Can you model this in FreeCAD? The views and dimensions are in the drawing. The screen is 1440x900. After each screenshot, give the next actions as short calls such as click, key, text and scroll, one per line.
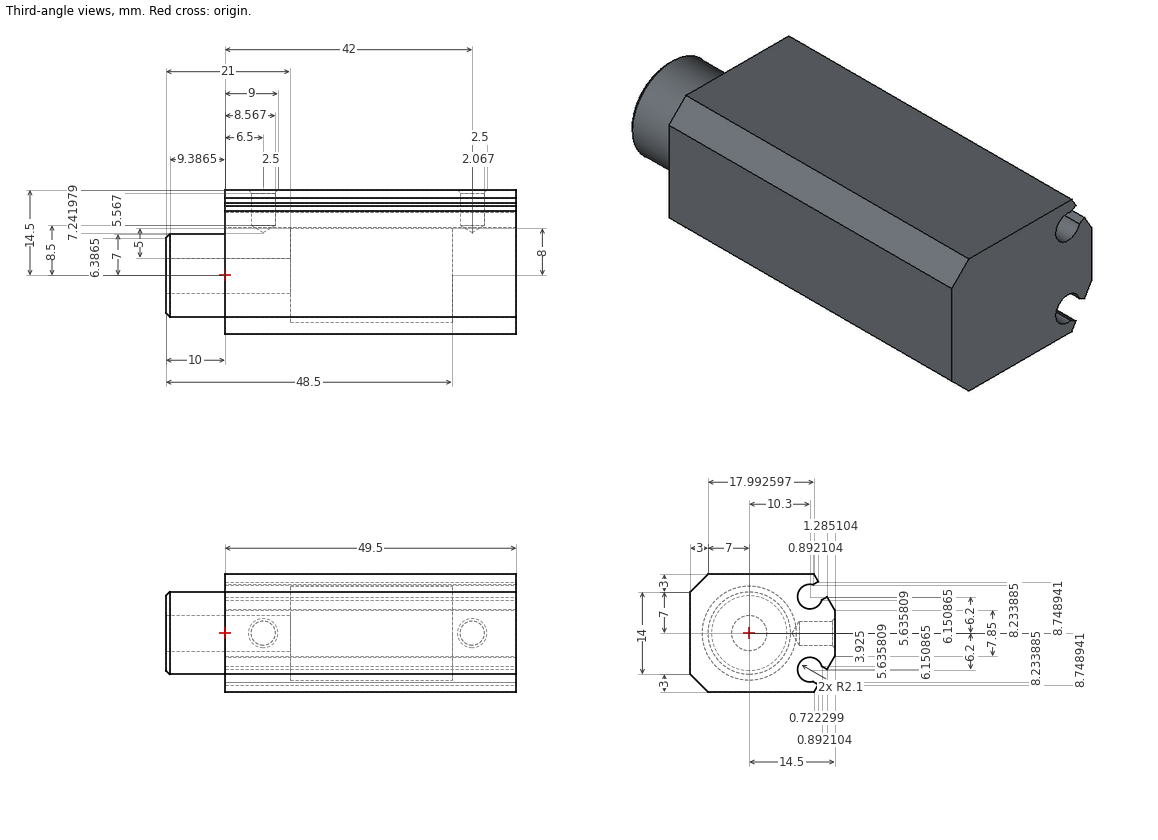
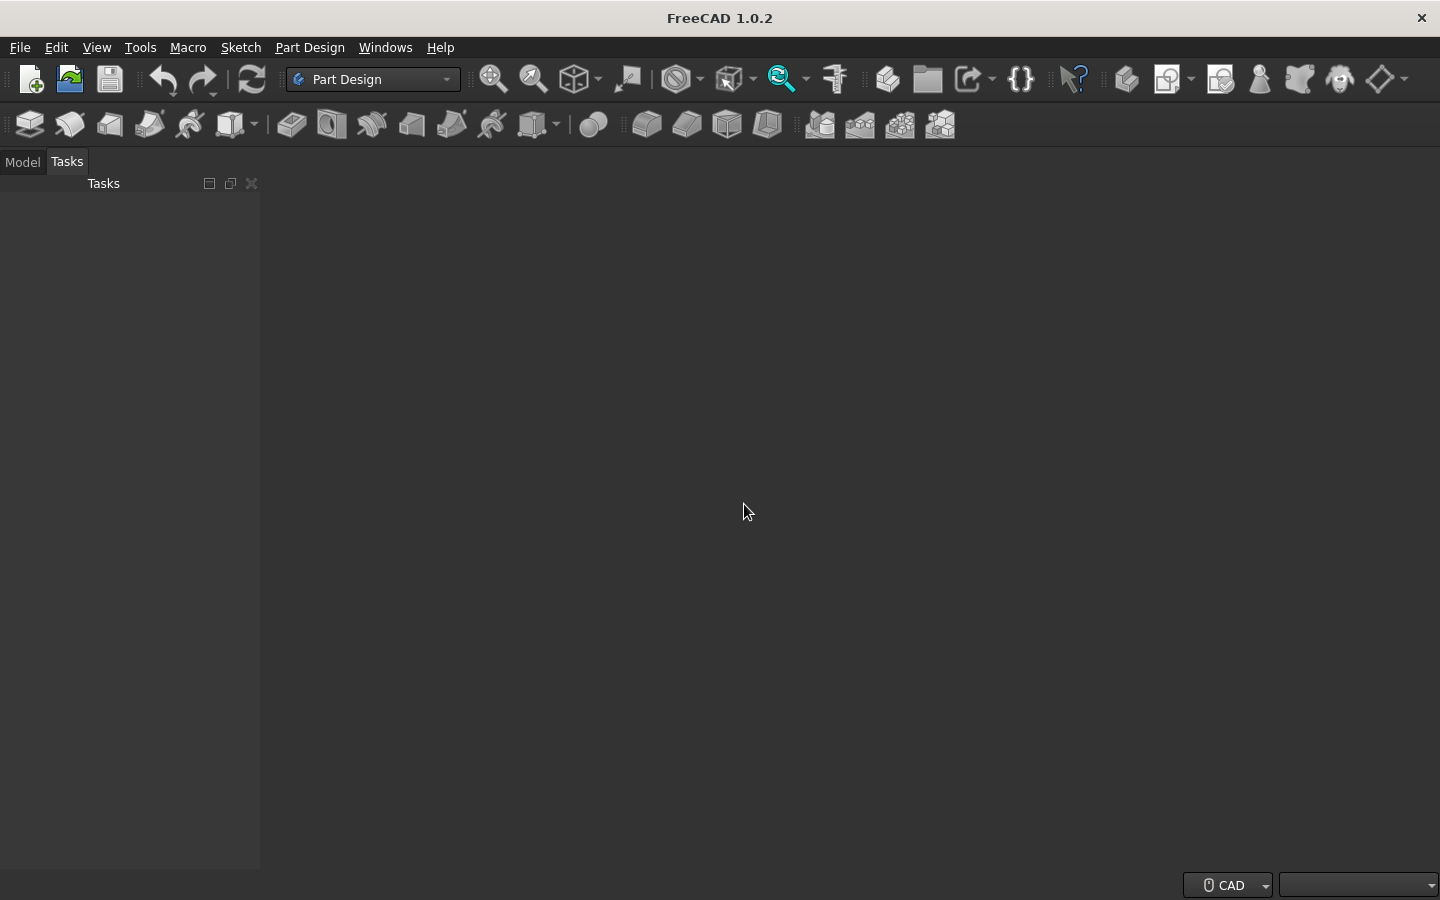
key(ctrl+n)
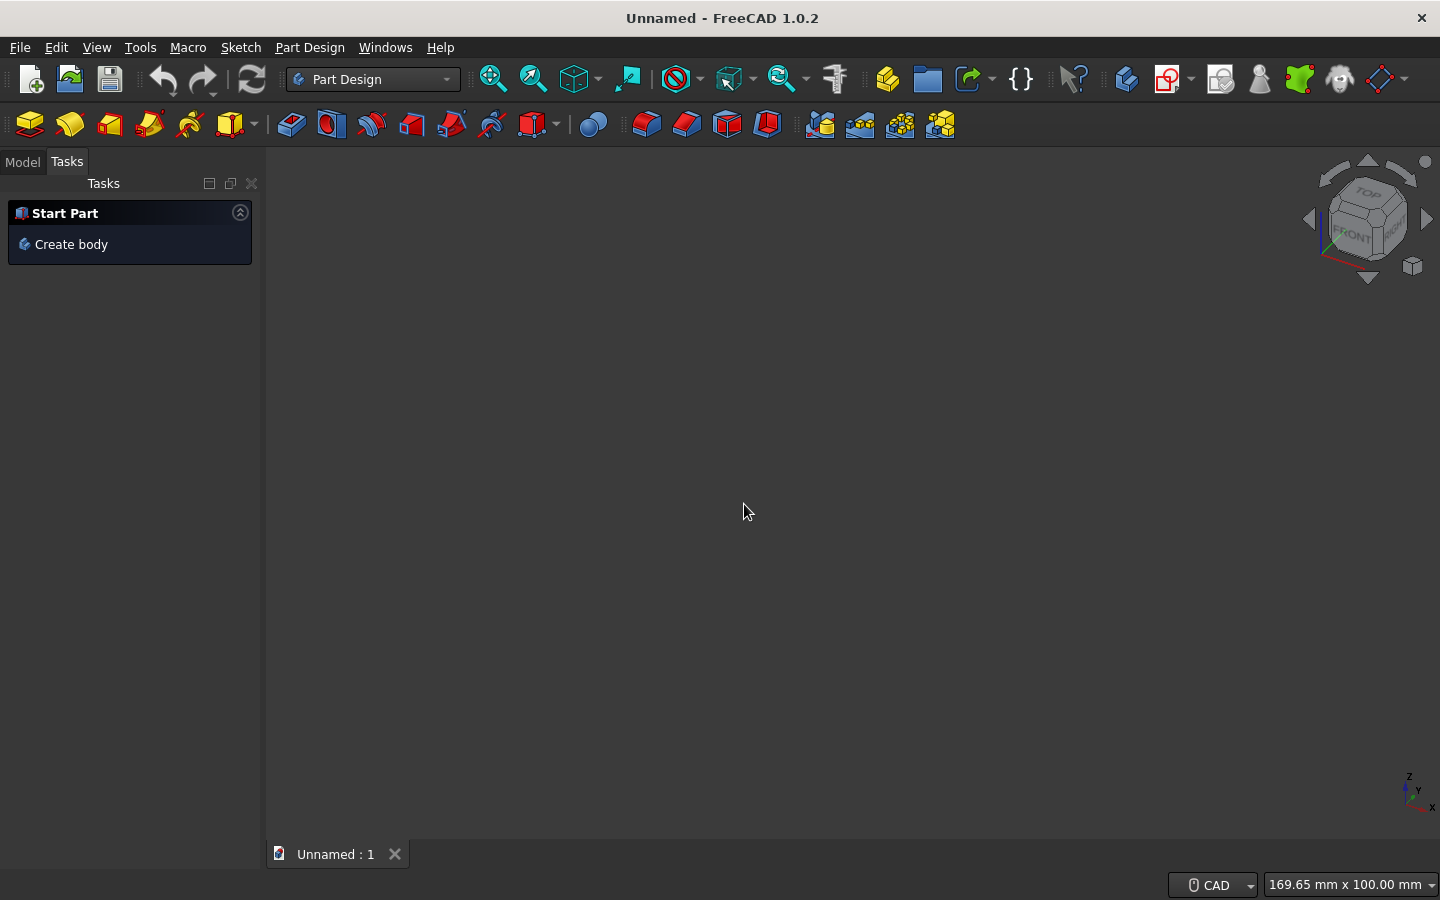
click(1168, 80)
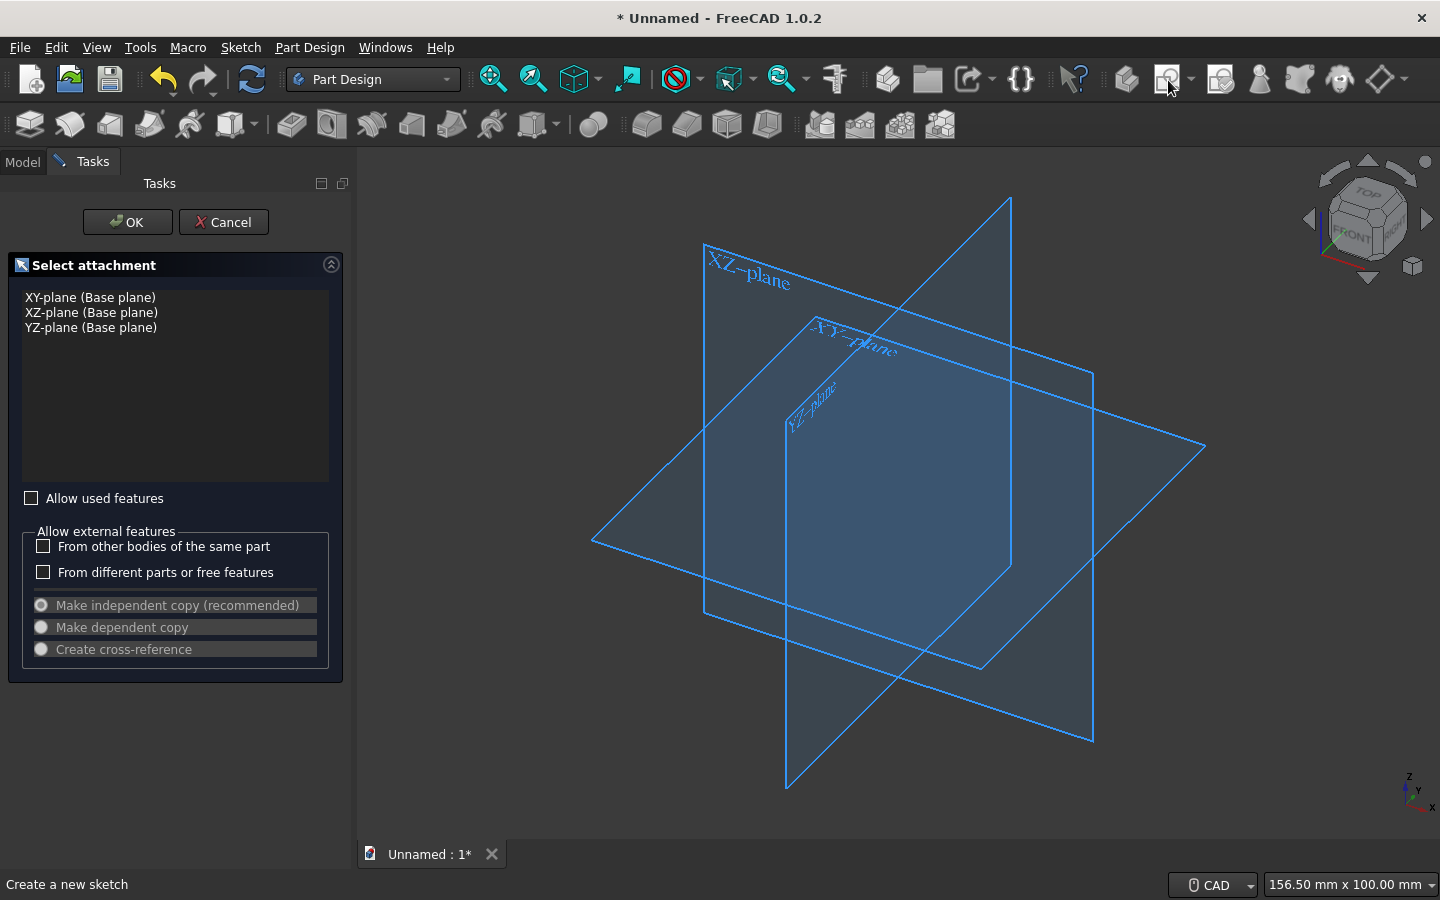
click(82, 328)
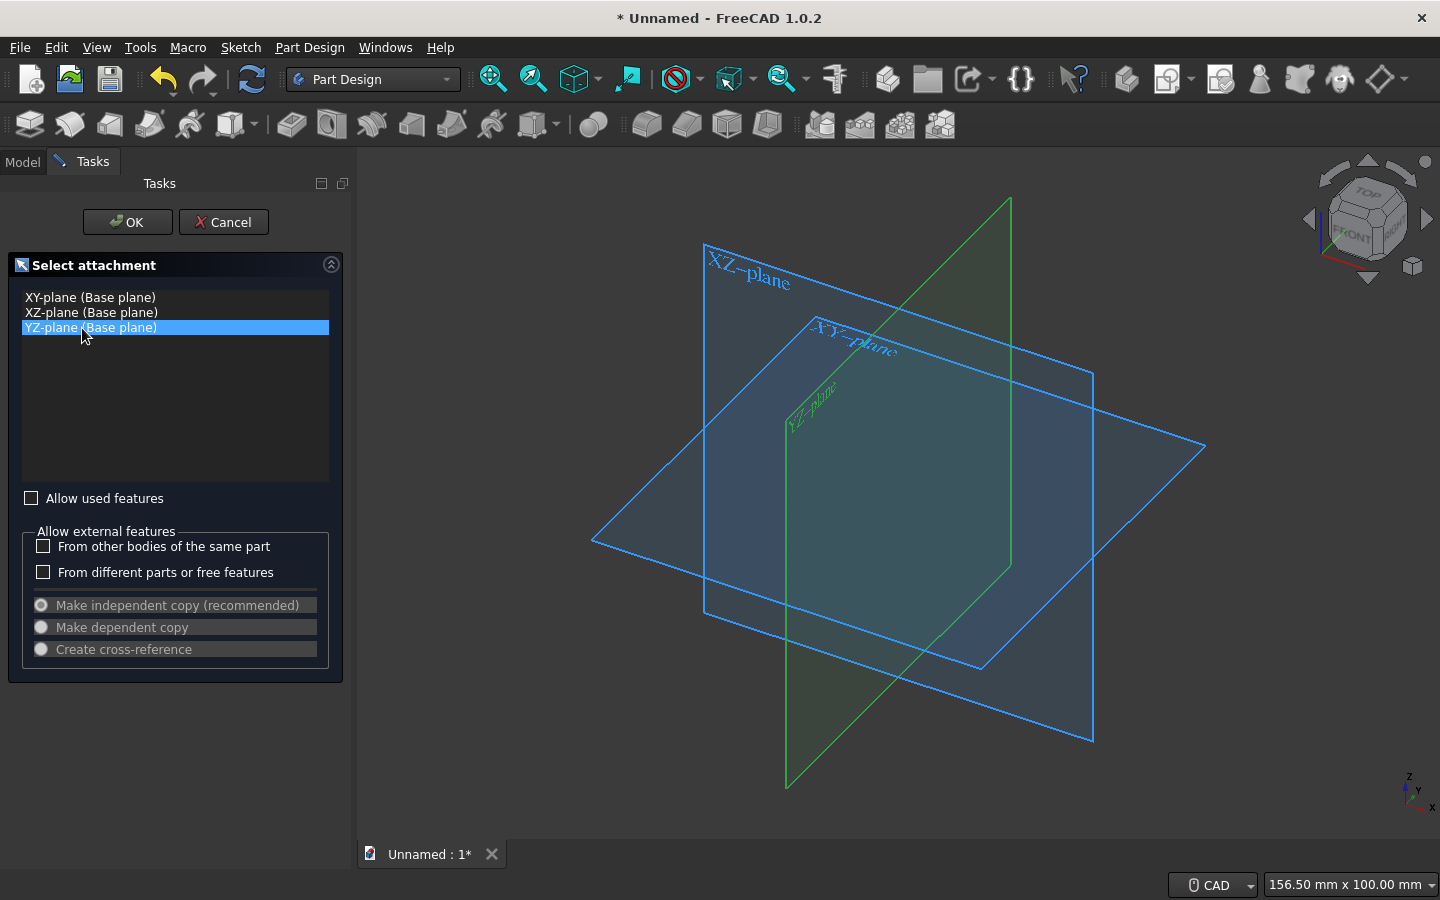
click(128, 222)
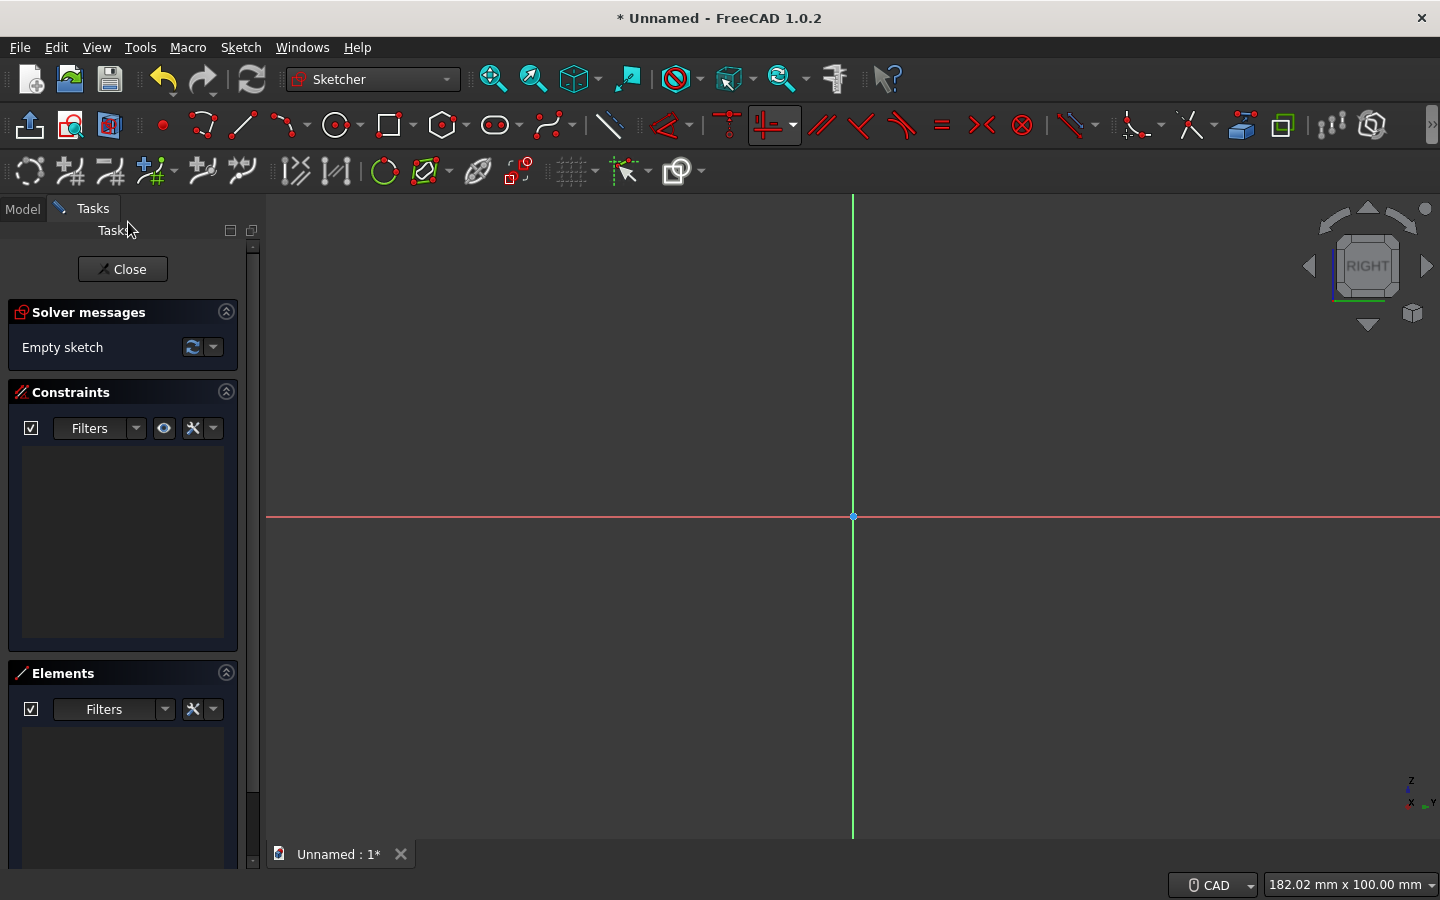
scroll(903, 516, up, 6)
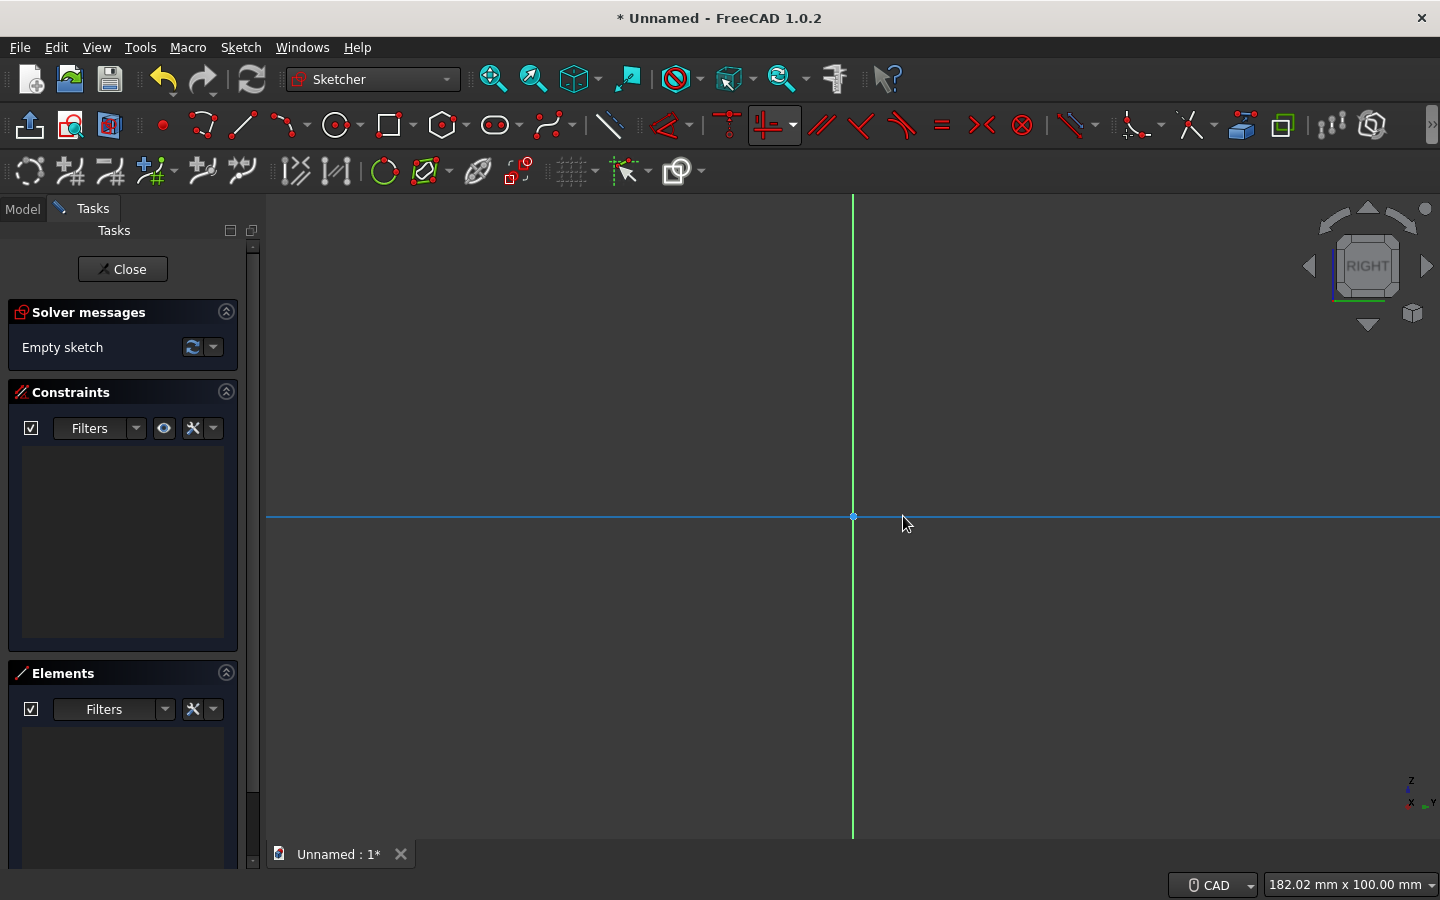
click(204, 126)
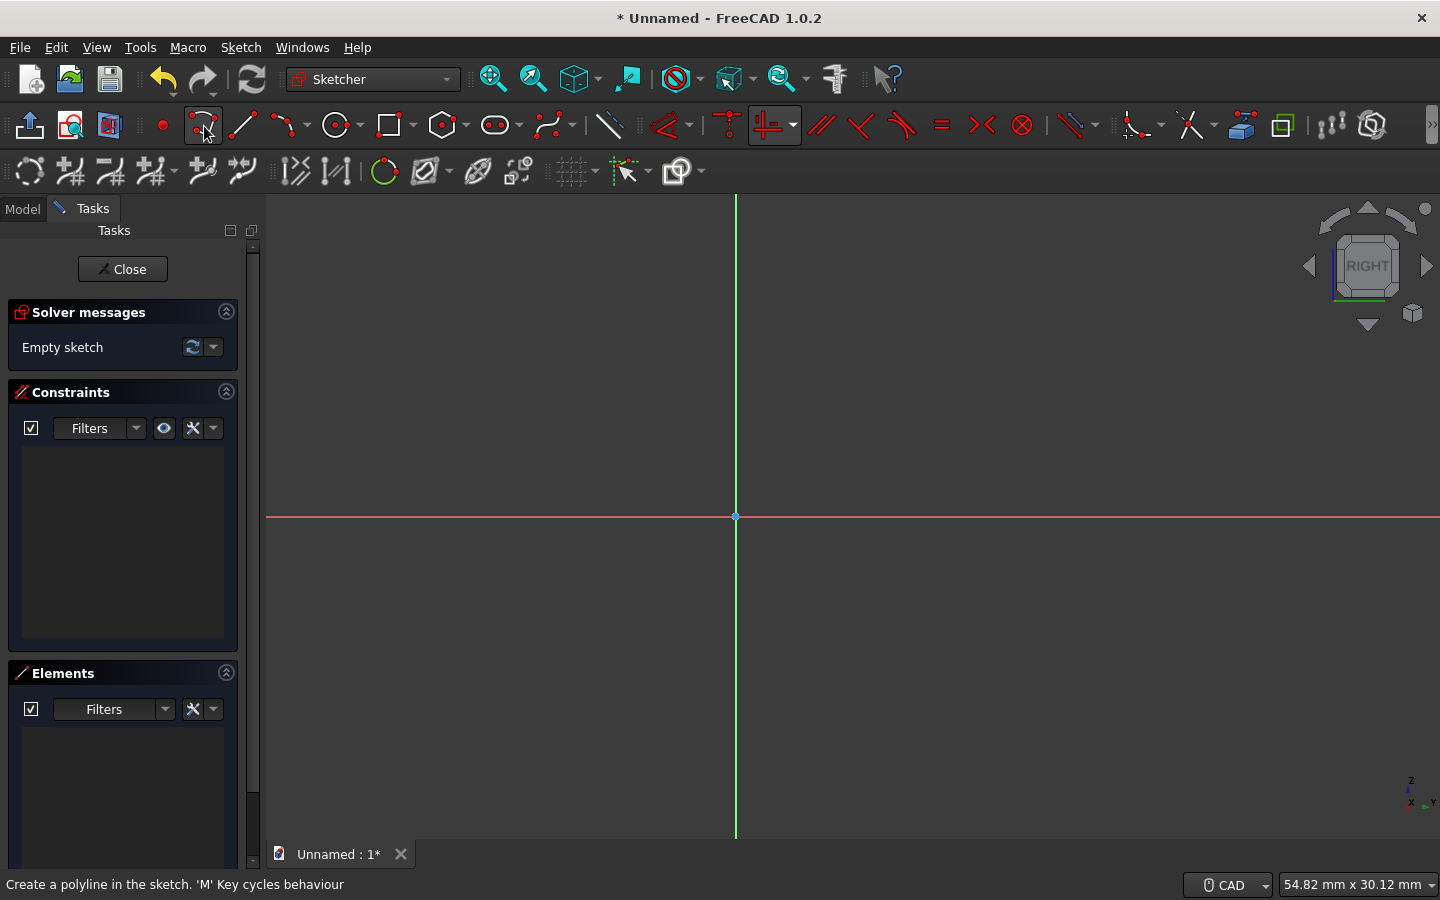
click(1000, 637)
click(1019, 648)
click(1046, 601)
click(1046, 432)
click(1019, 385)
click(1000, 396)
right_click(1000, 396)